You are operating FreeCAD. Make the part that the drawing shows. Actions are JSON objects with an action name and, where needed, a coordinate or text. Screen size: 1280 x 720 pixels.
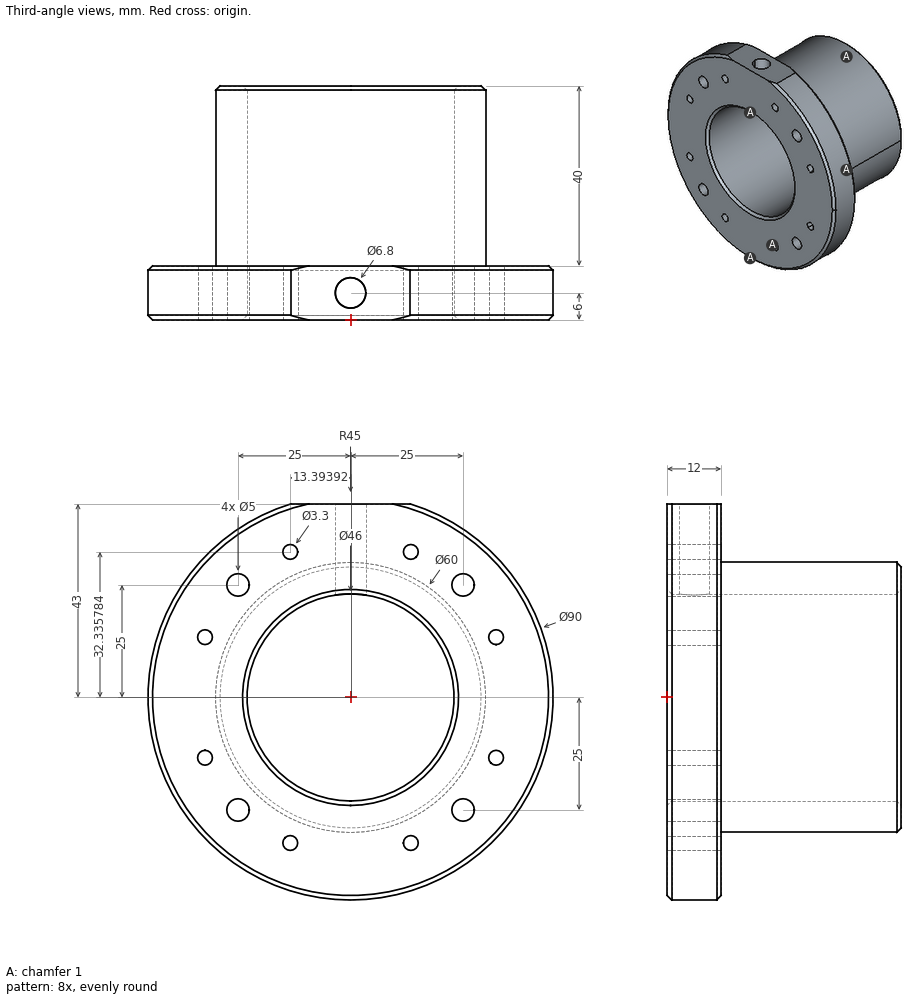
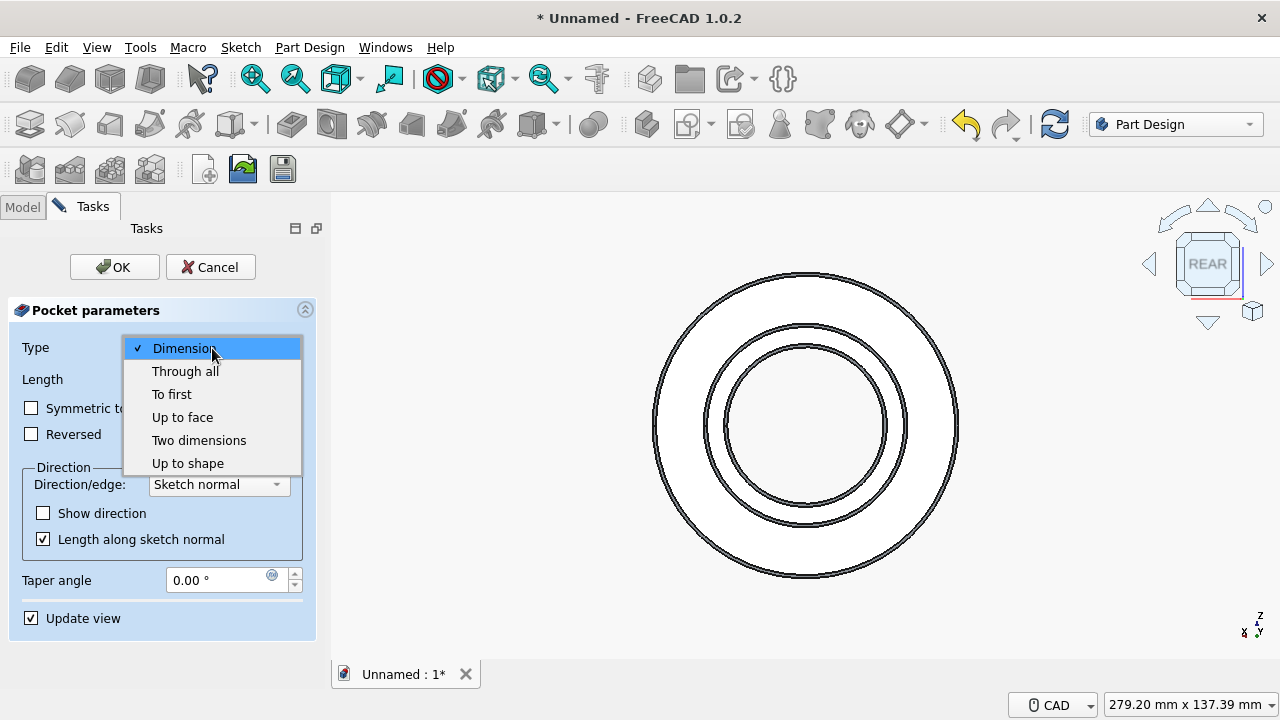
{"action": "left_click", "coordinate": [212, 372]}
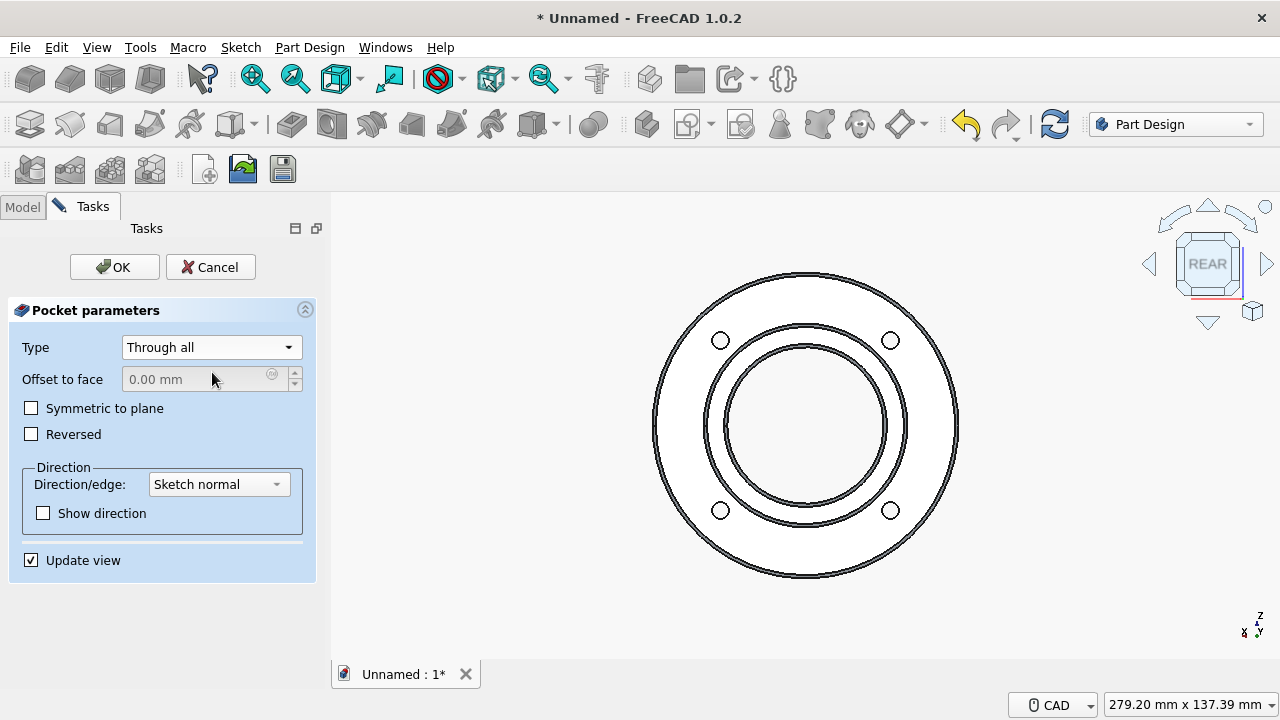
{"action": "left_click", "coordinate": [115, 267]}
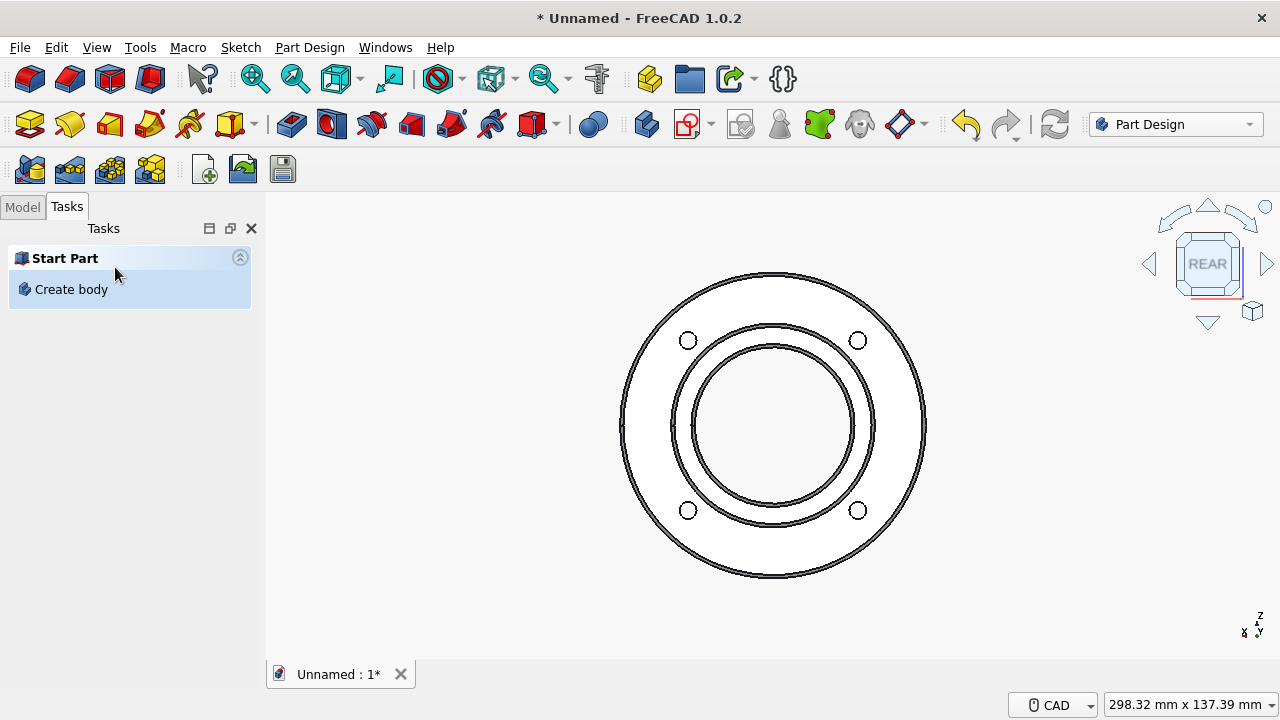
{"action": "left_click", "coordinate": [688, 124]}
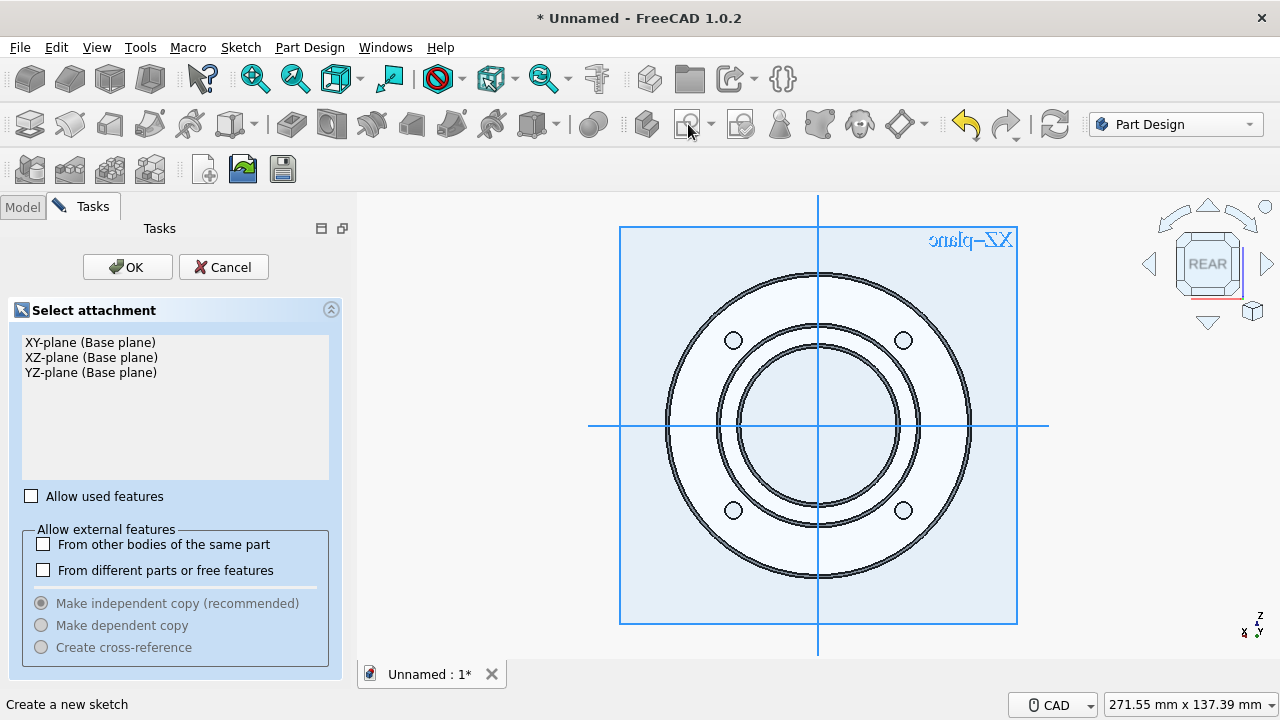
{"action": "left_click", "coordinate": [82, 358]}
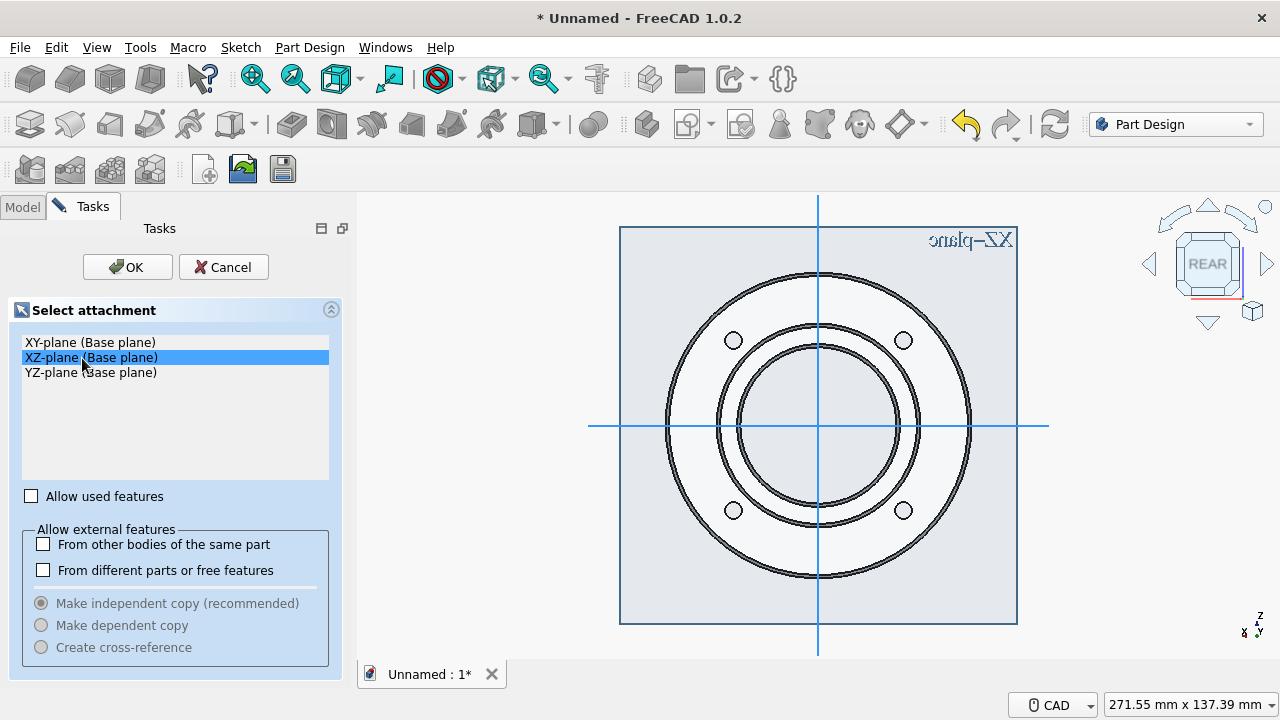
{"action": "left_click", "coordinate": [128, 267]}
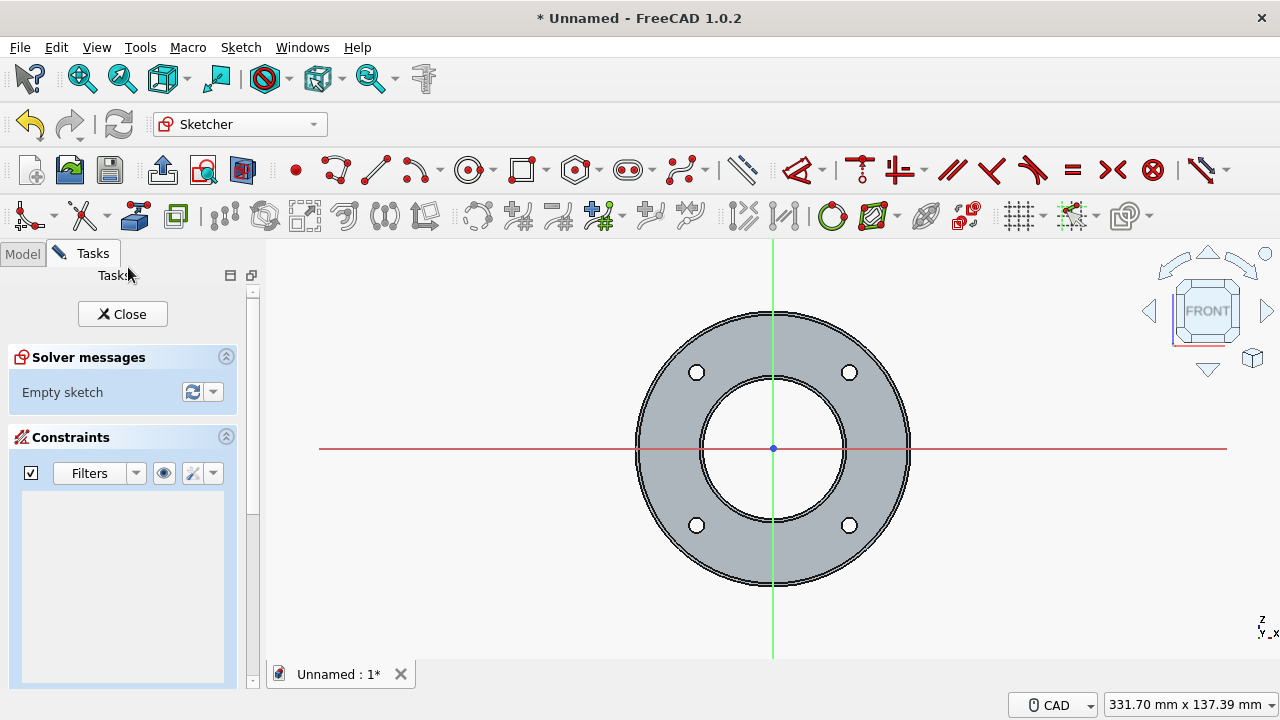
{"action": "scroll", "coordinate": [733, 345], "scroll_direction": "up", "scroll_amount": 15}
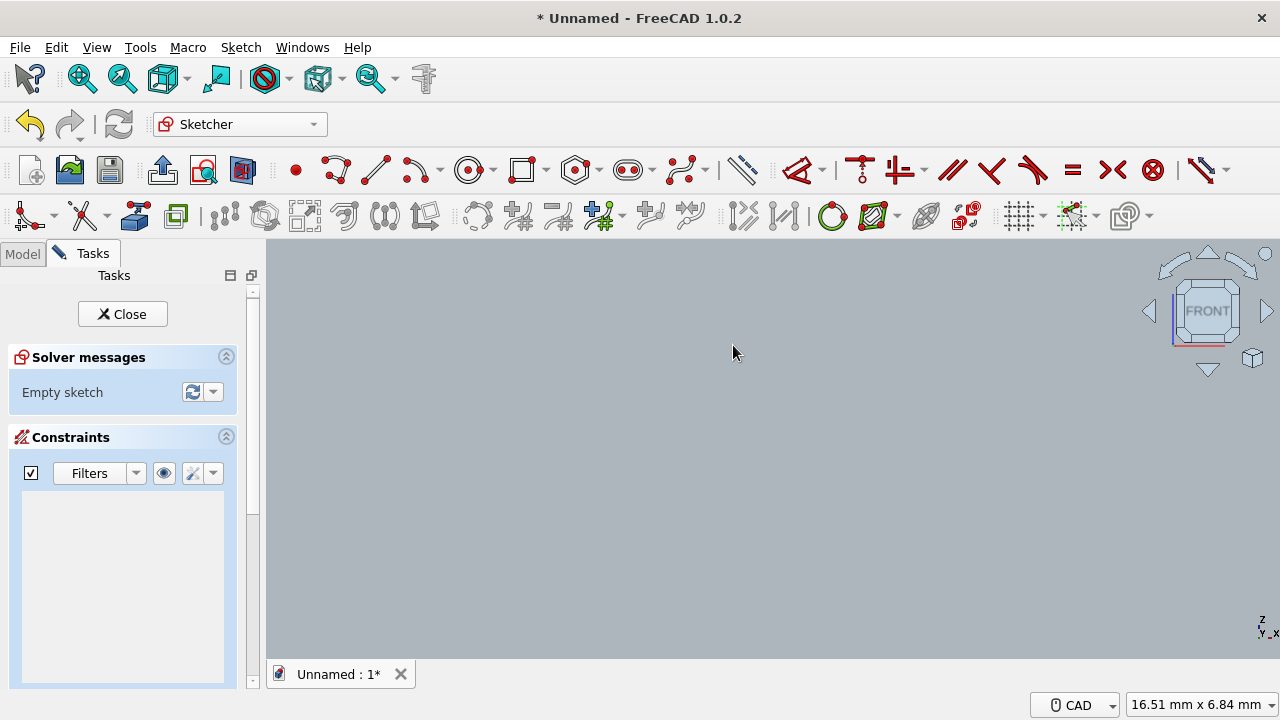
{"action": "left_click", "coordinate": [470, 170]}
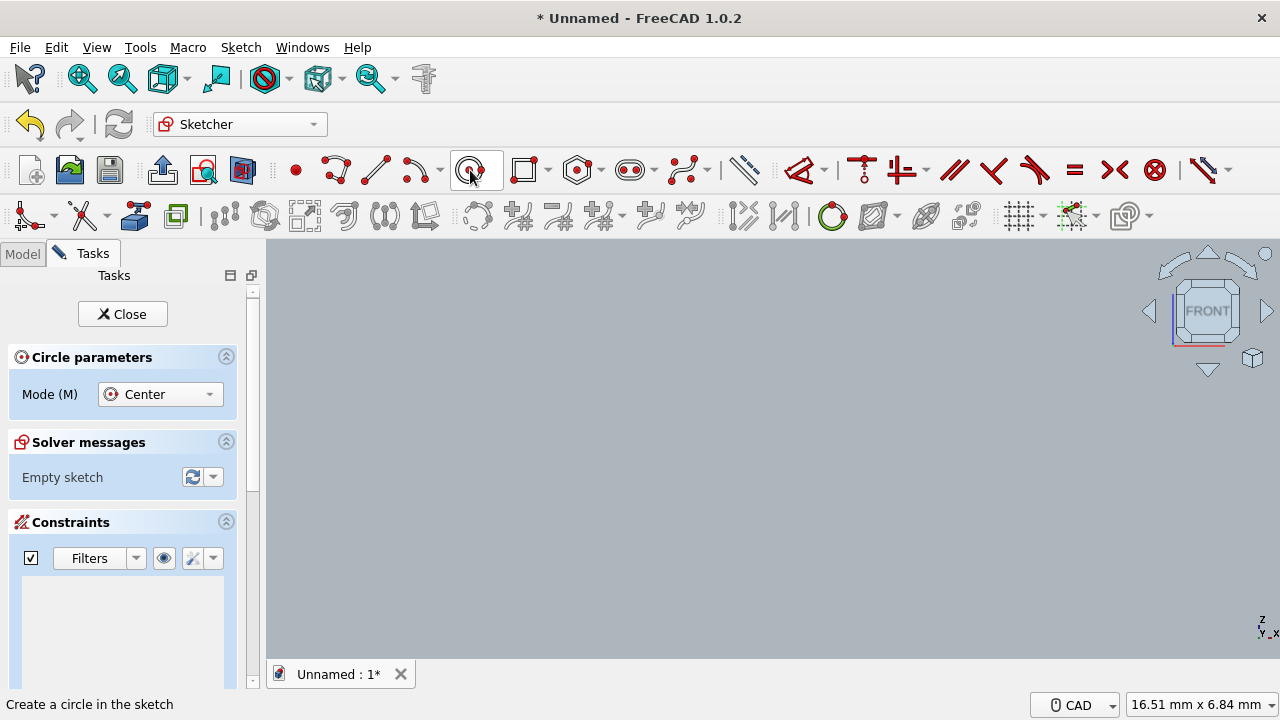
{"action": "left_click", "coordinate": [705, 444]}
{"action": "left_click", "coordinate": [777, 372]}
{"action": "key", "text": "Escape"}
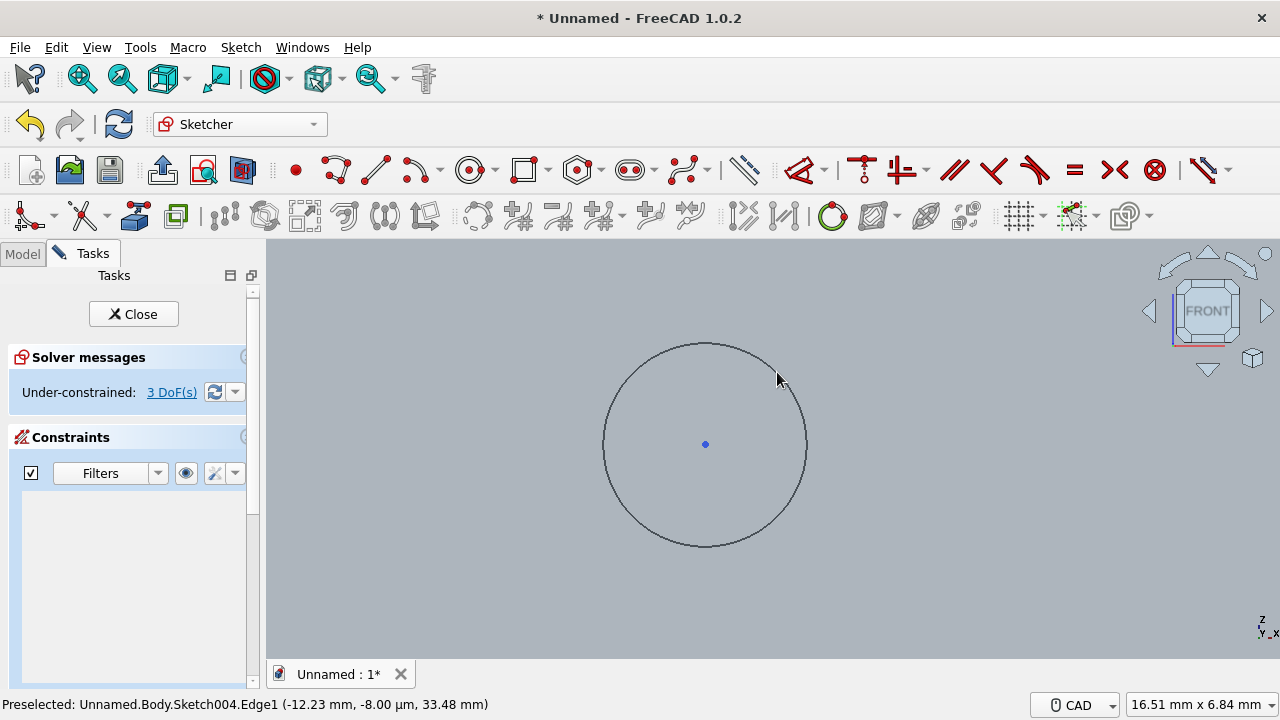
{"action": "key", "text": "d"}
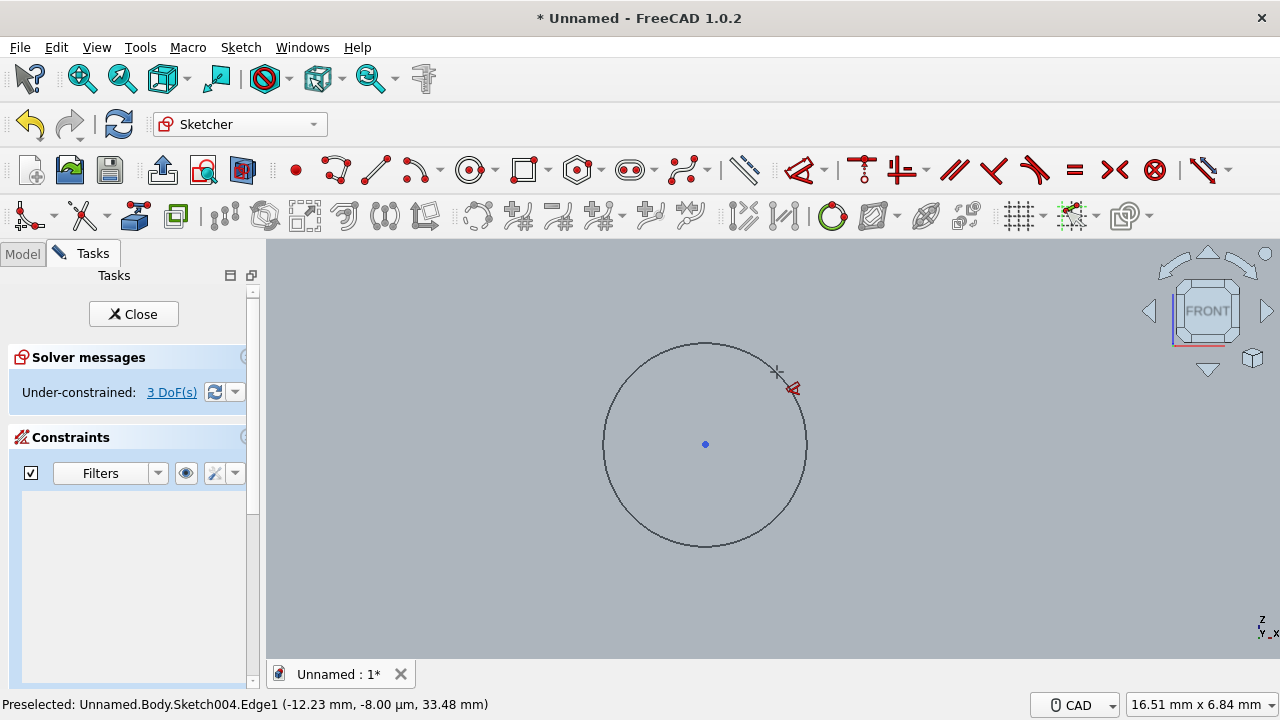
{"action": "left_click", "coordinate": [777, 373]}
{"action": "left_click", "coordinate": [800, 350]}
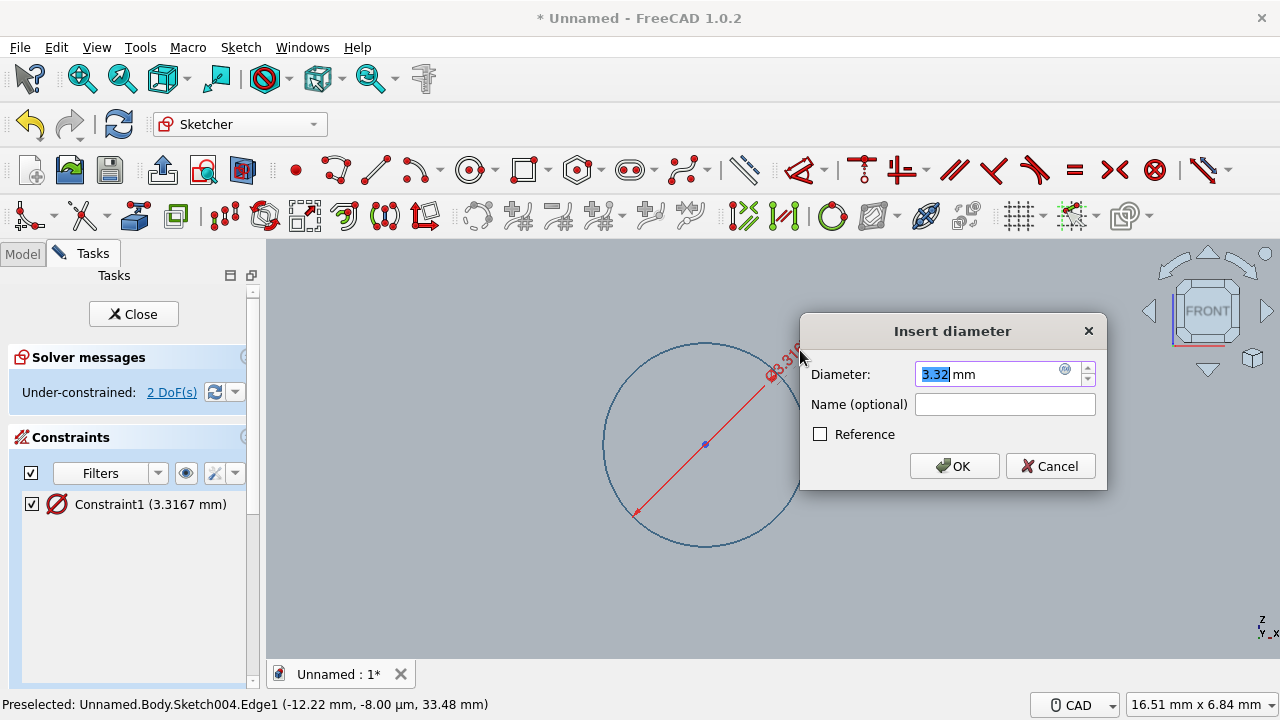
{"action": "type", "text": "3.3"}
{"action": "key", "text": "Return"}